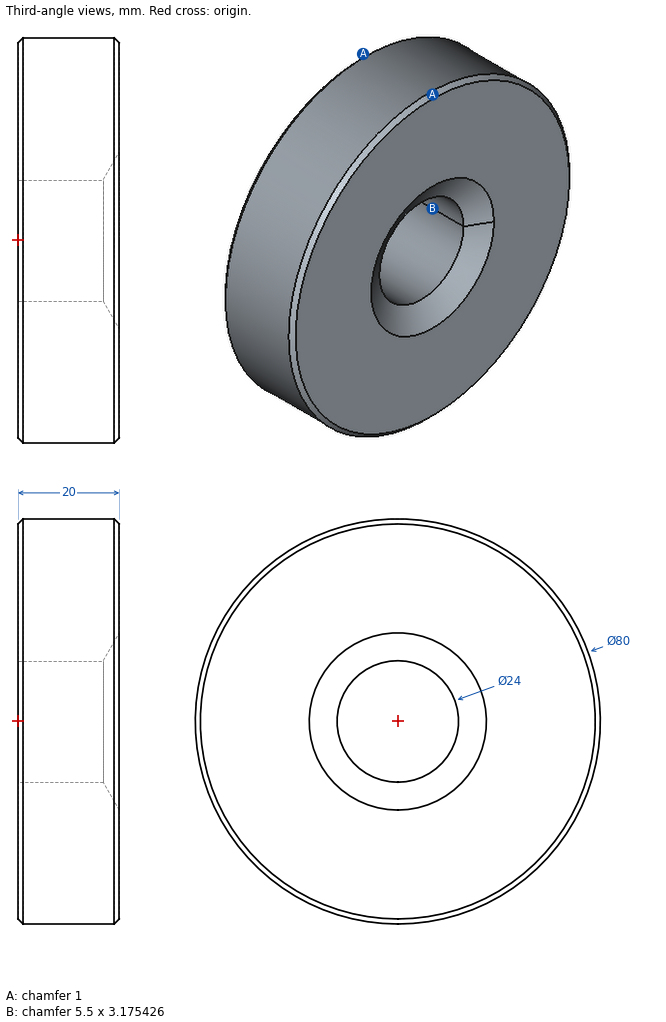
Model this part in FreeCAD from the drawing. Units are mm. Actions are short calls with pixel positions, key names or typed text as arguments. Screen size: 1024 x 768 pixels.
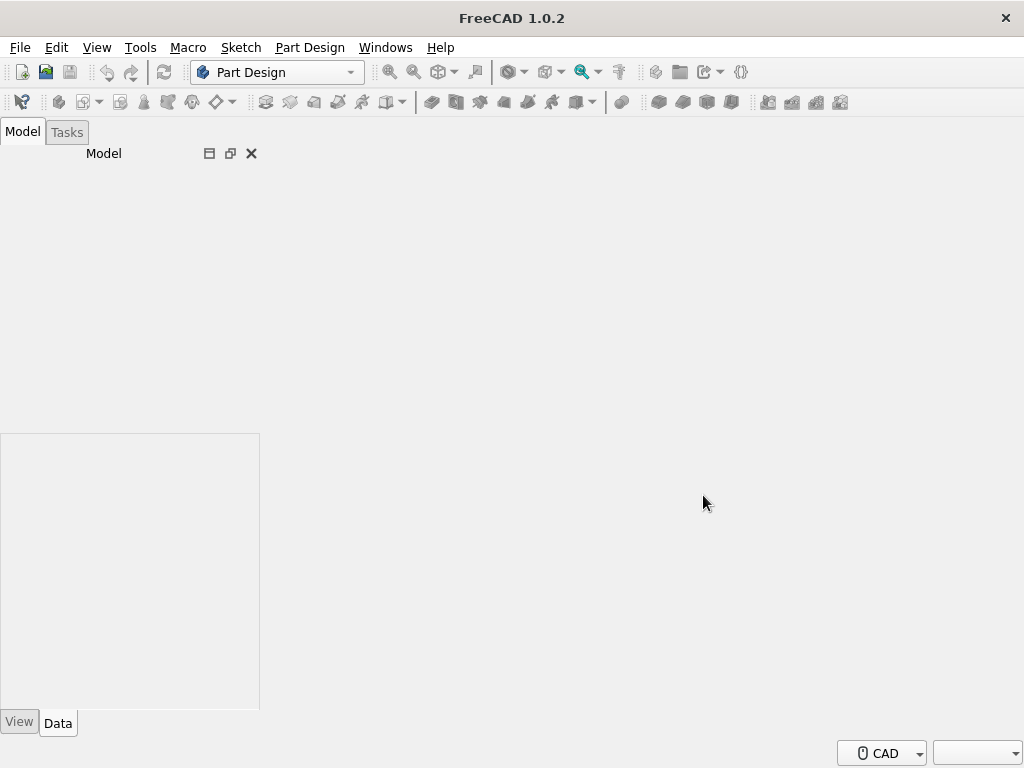
click(22, 72)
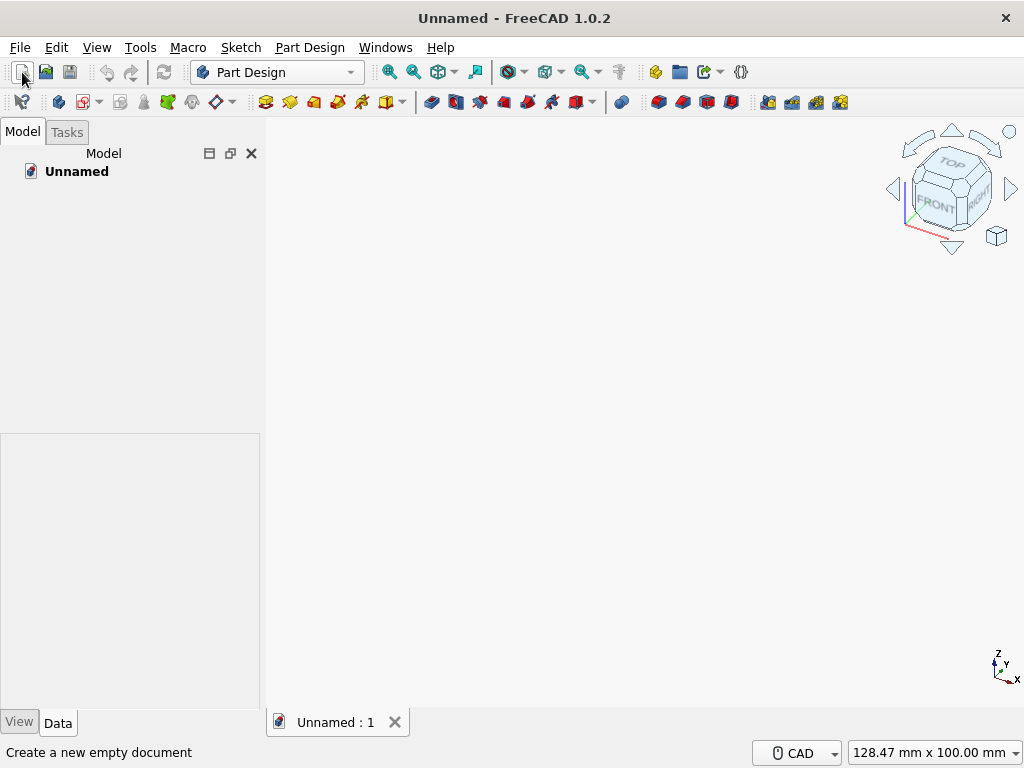
click(84, 102)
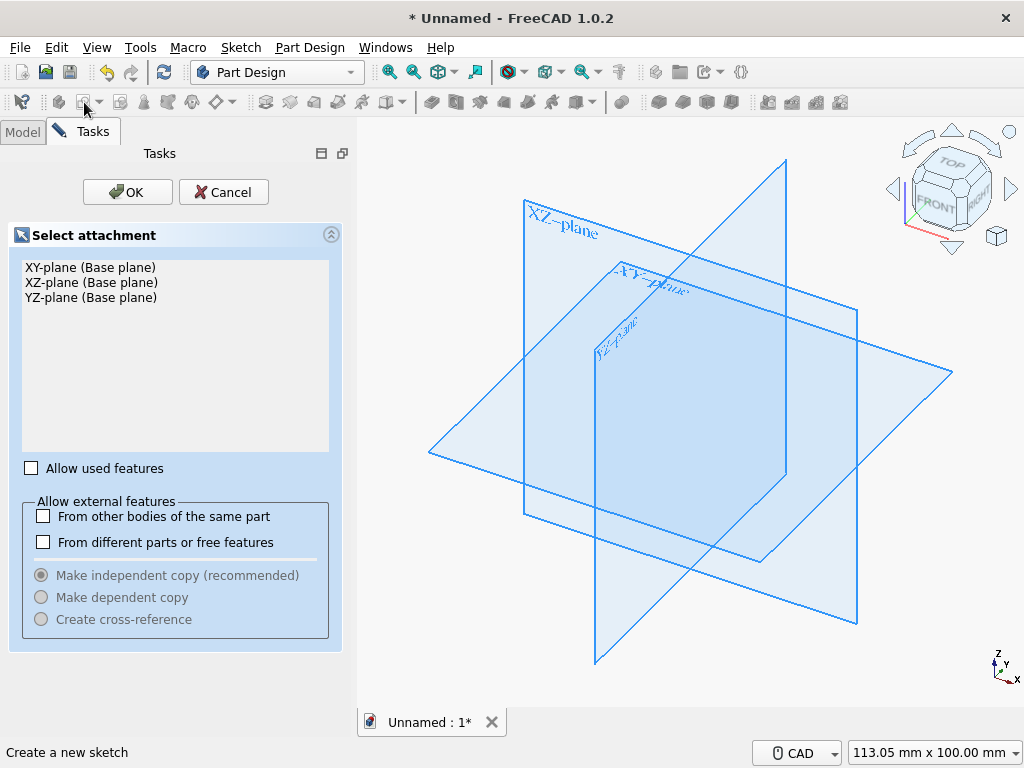
click(82, 298)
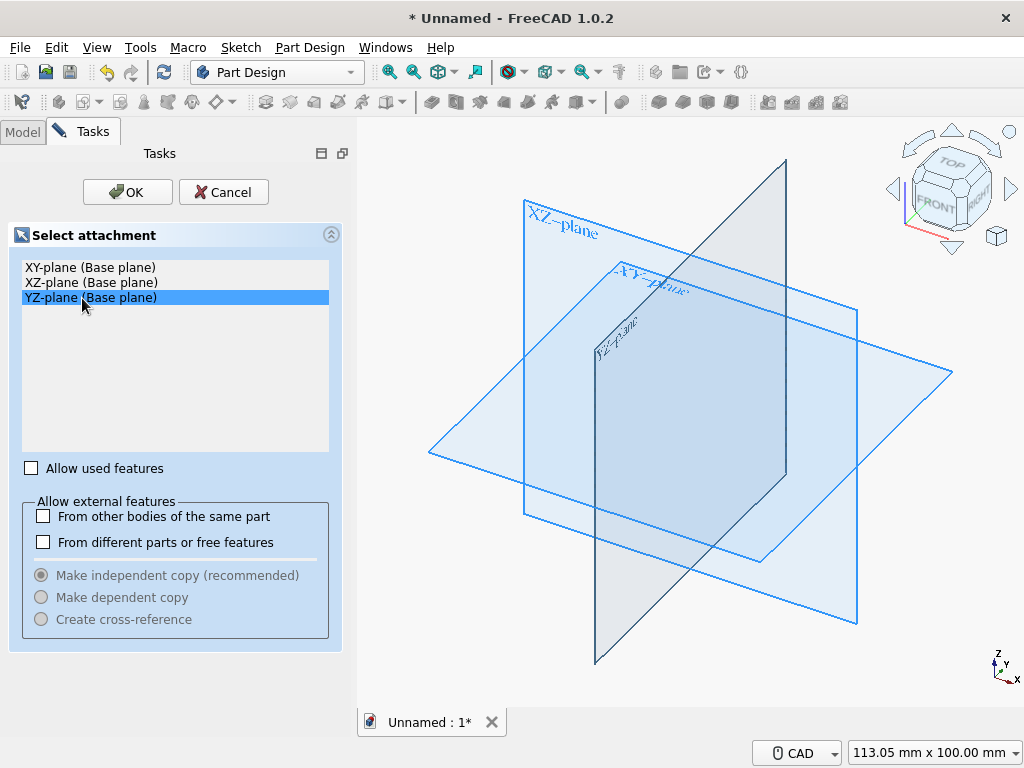
click(128, 192)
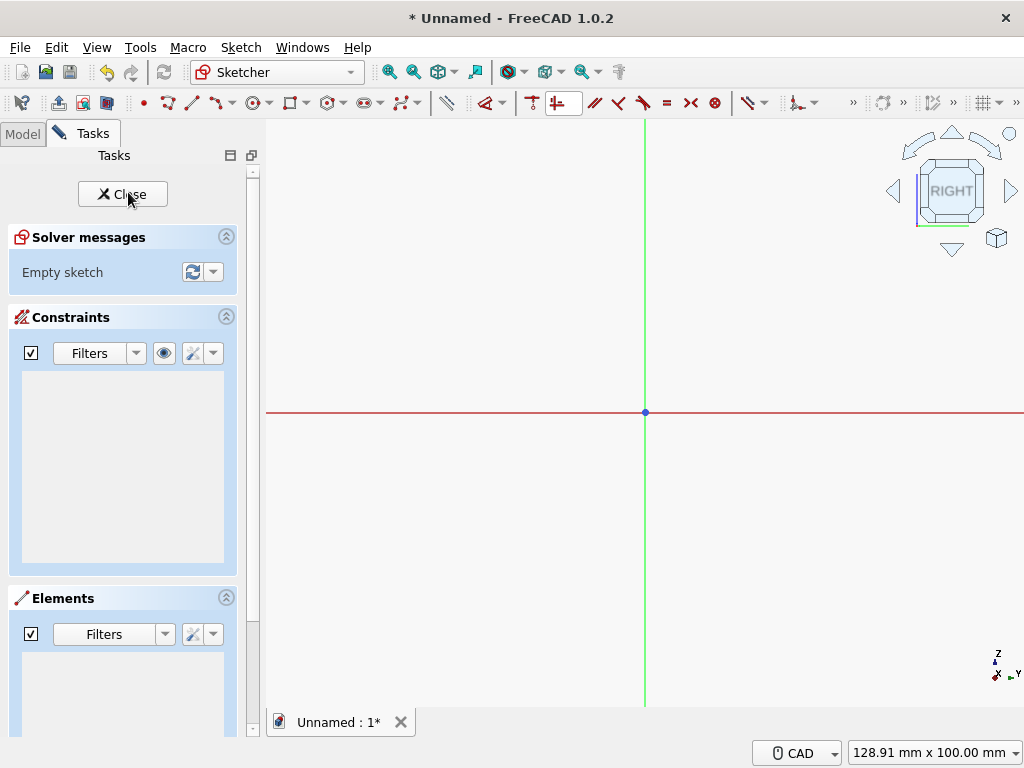
scroll(294, 413, down, 1)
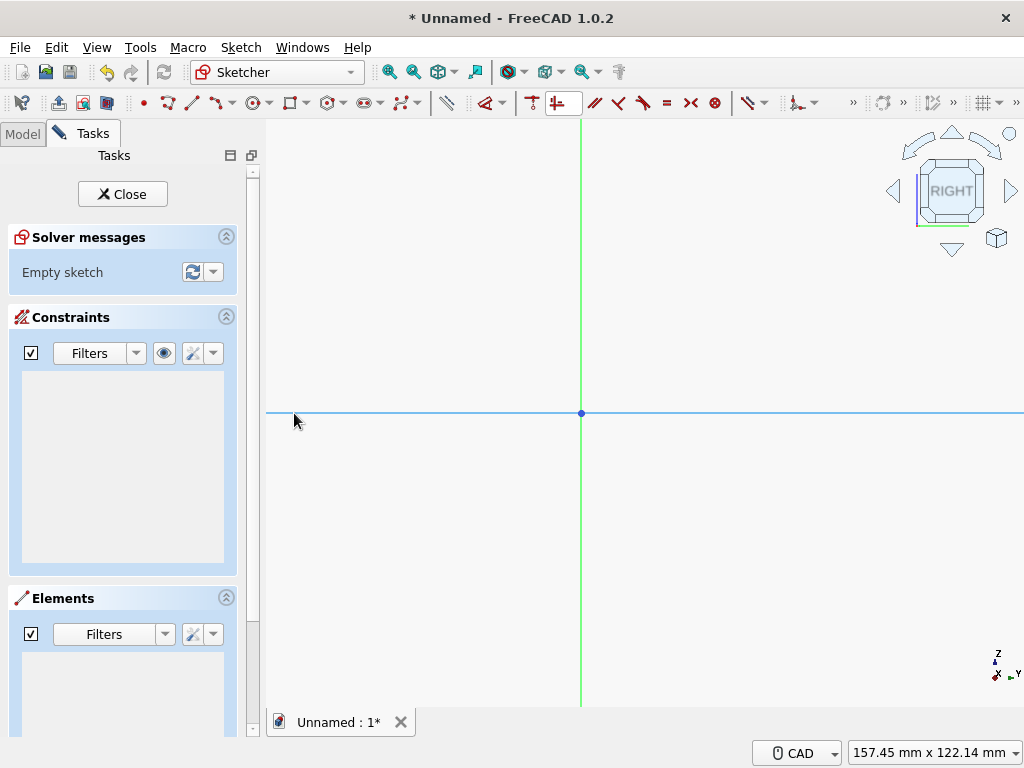
click(254, 104)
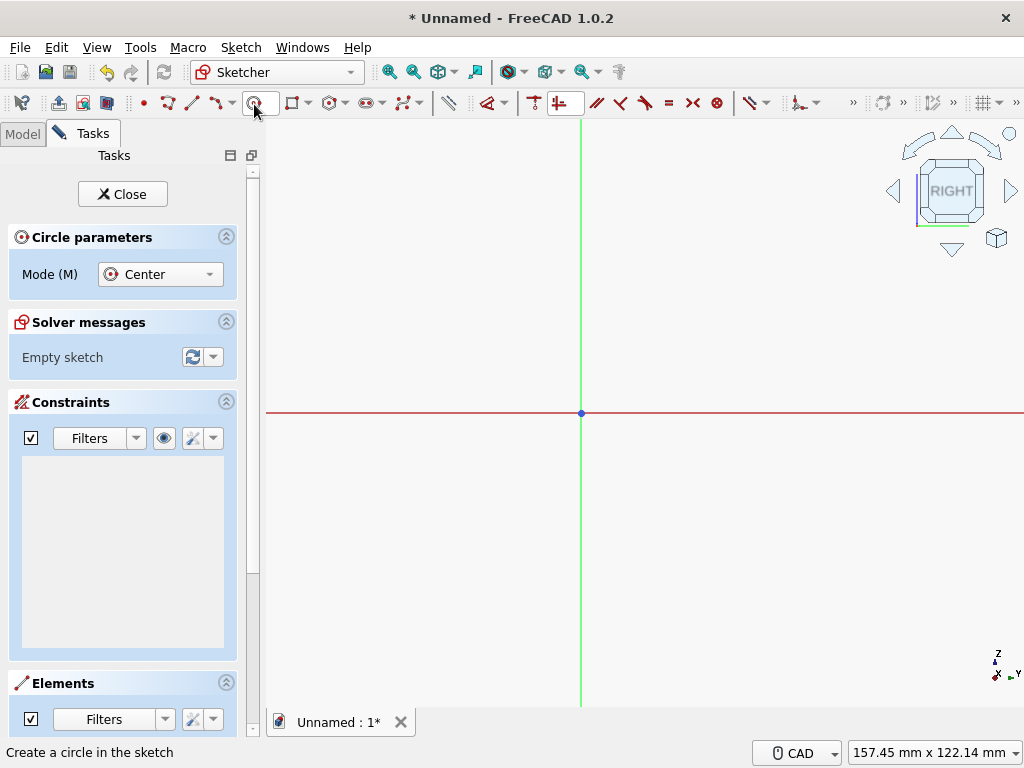
click(581, 413)
click(718, 277)
key(Escape)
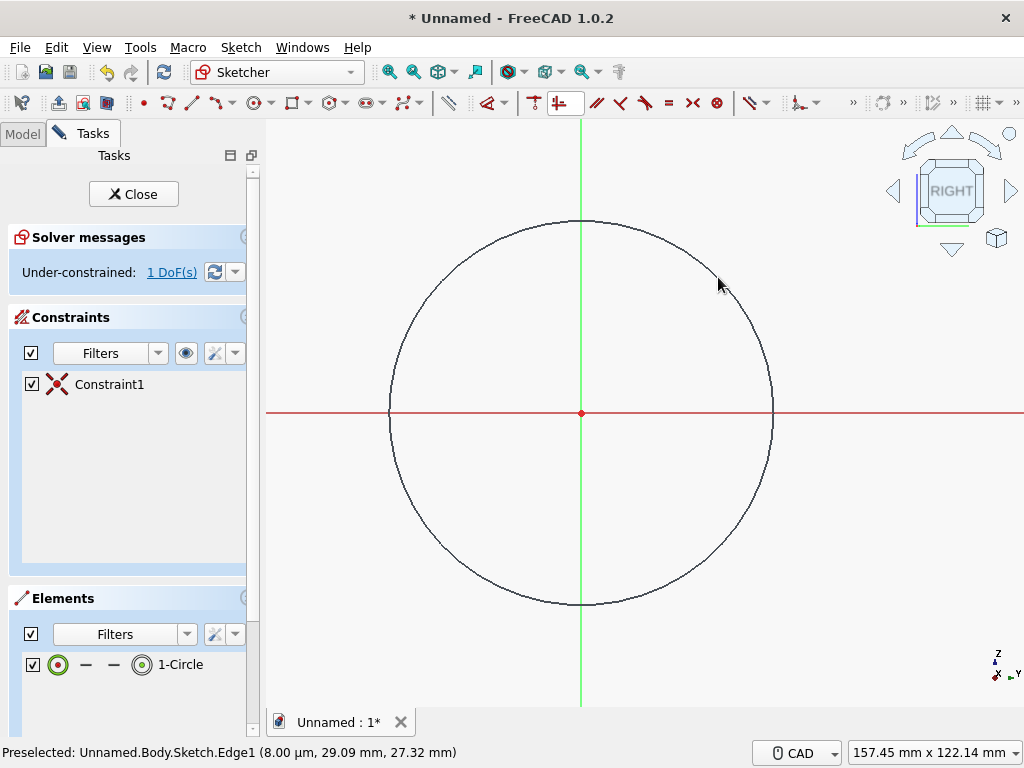
click(717, 277)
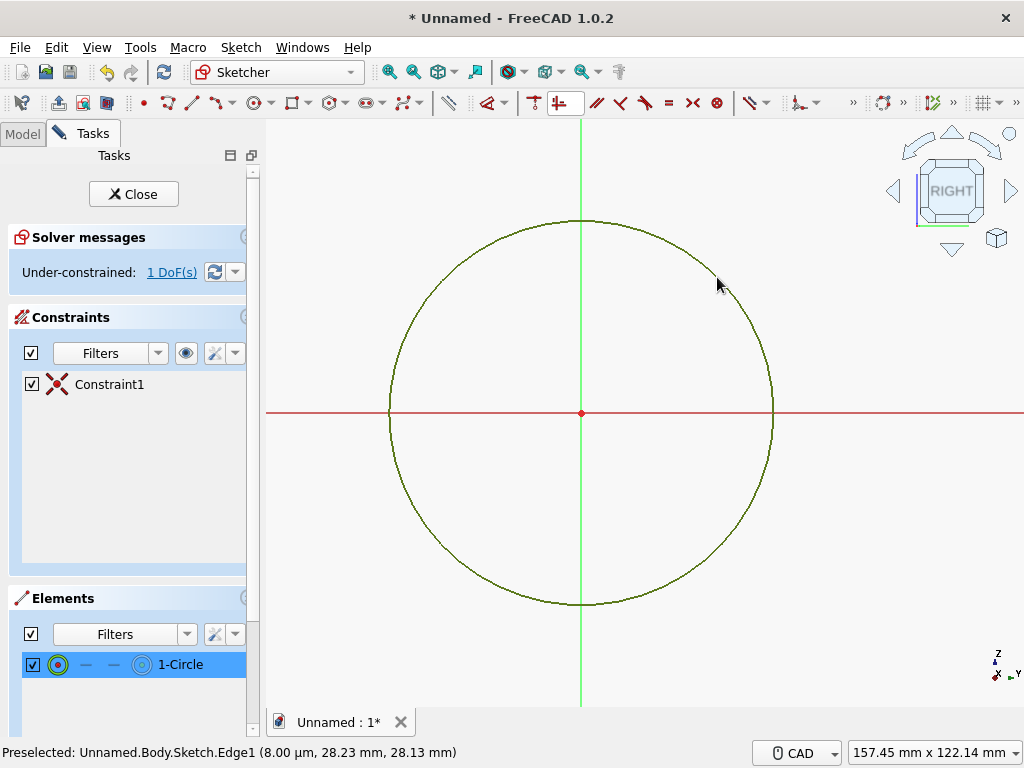
click(506, 104)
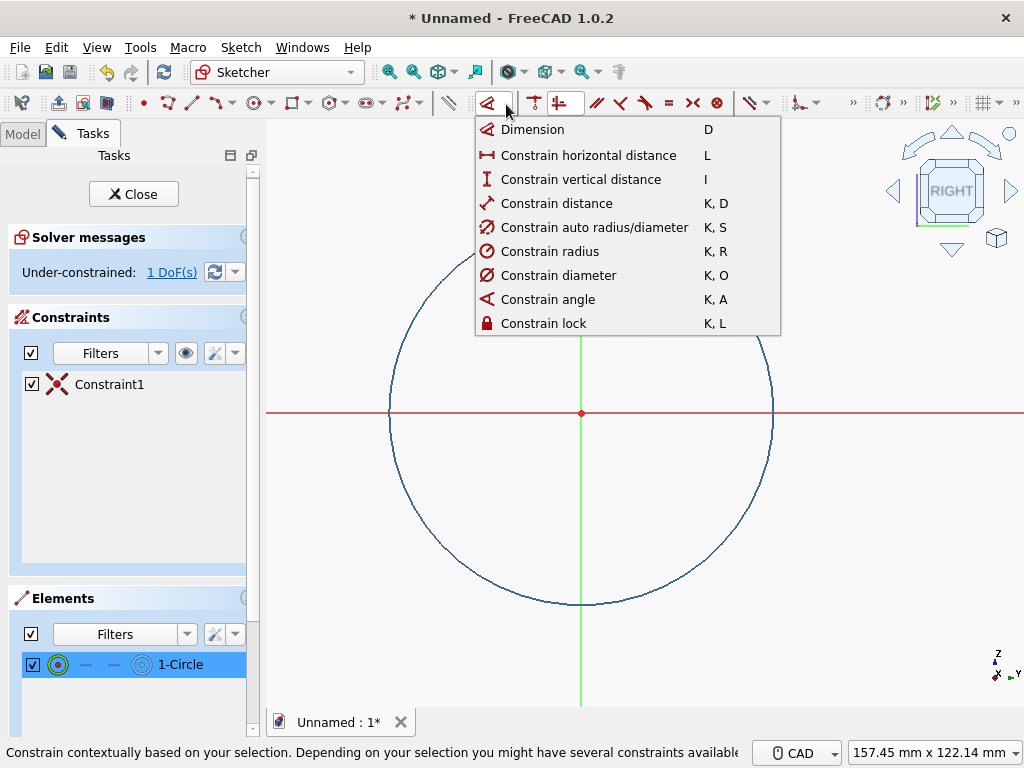
click(628, 275)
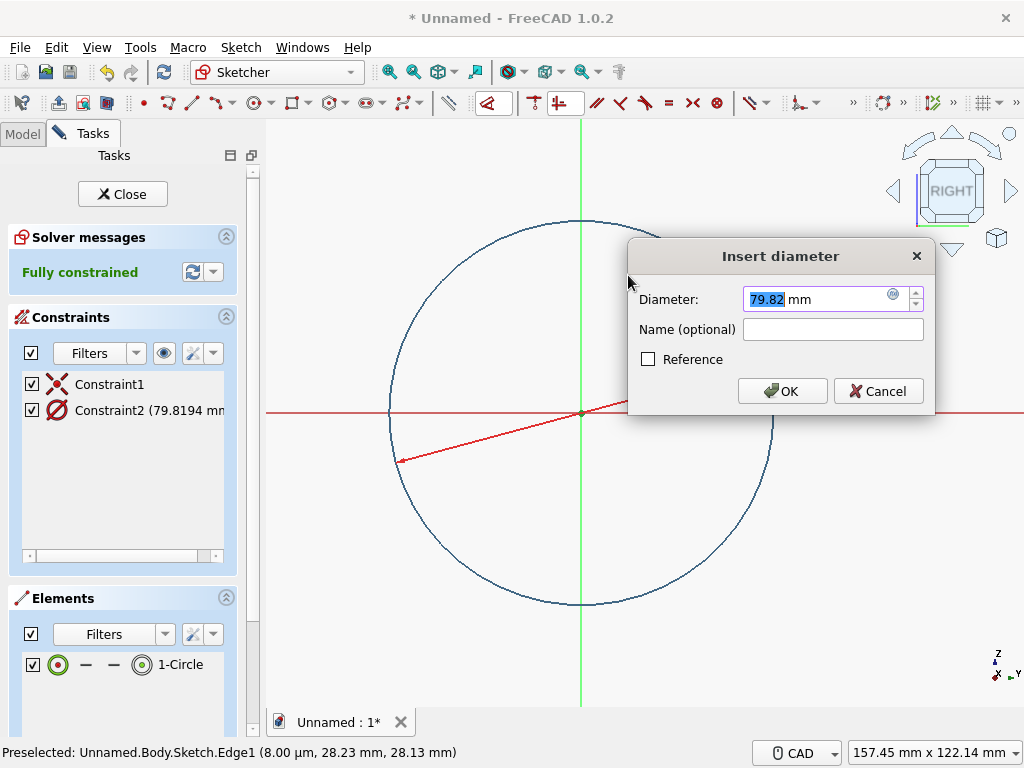
text(80)
key(Return)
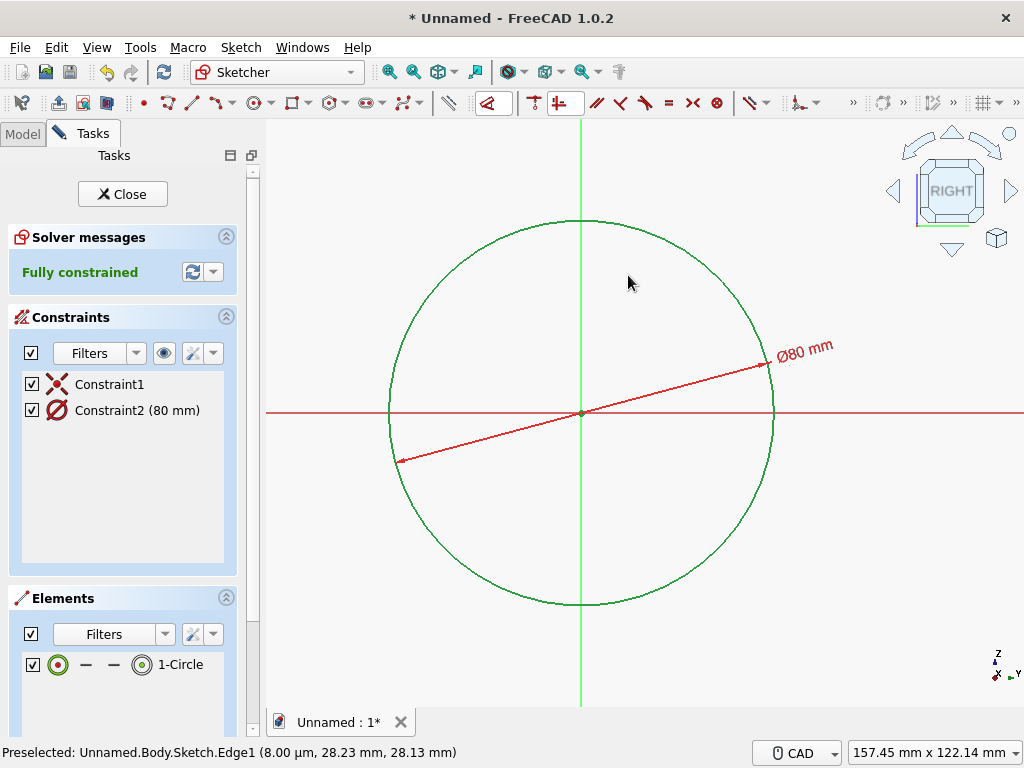
click(123, 194)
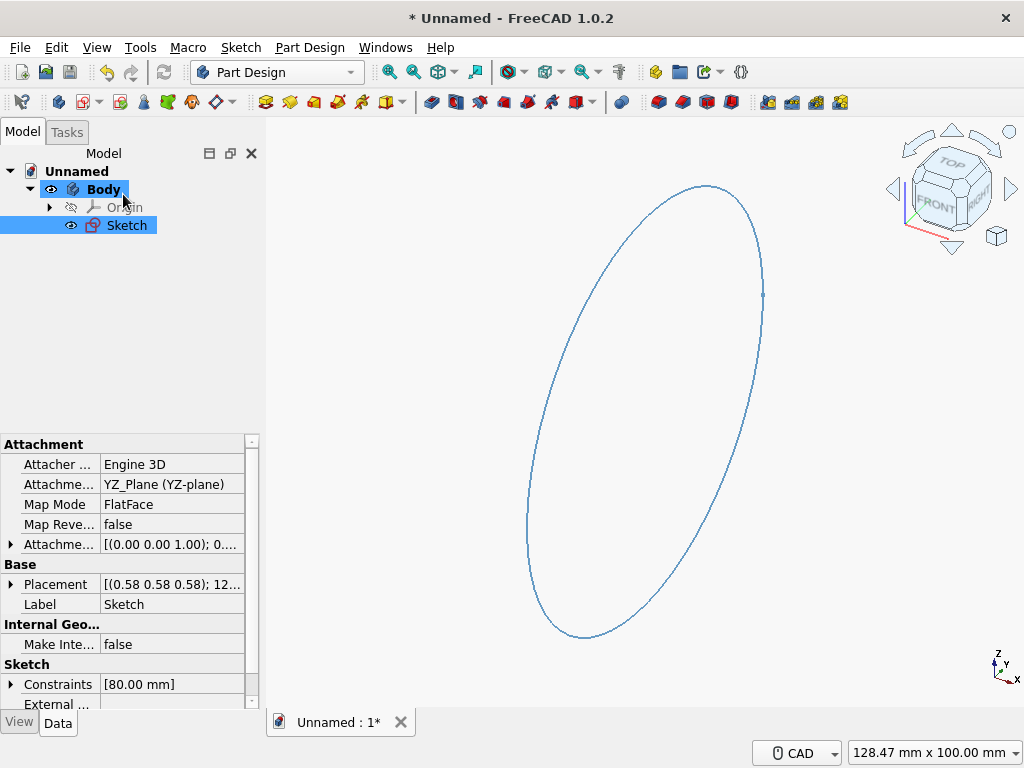
click(266, 102)